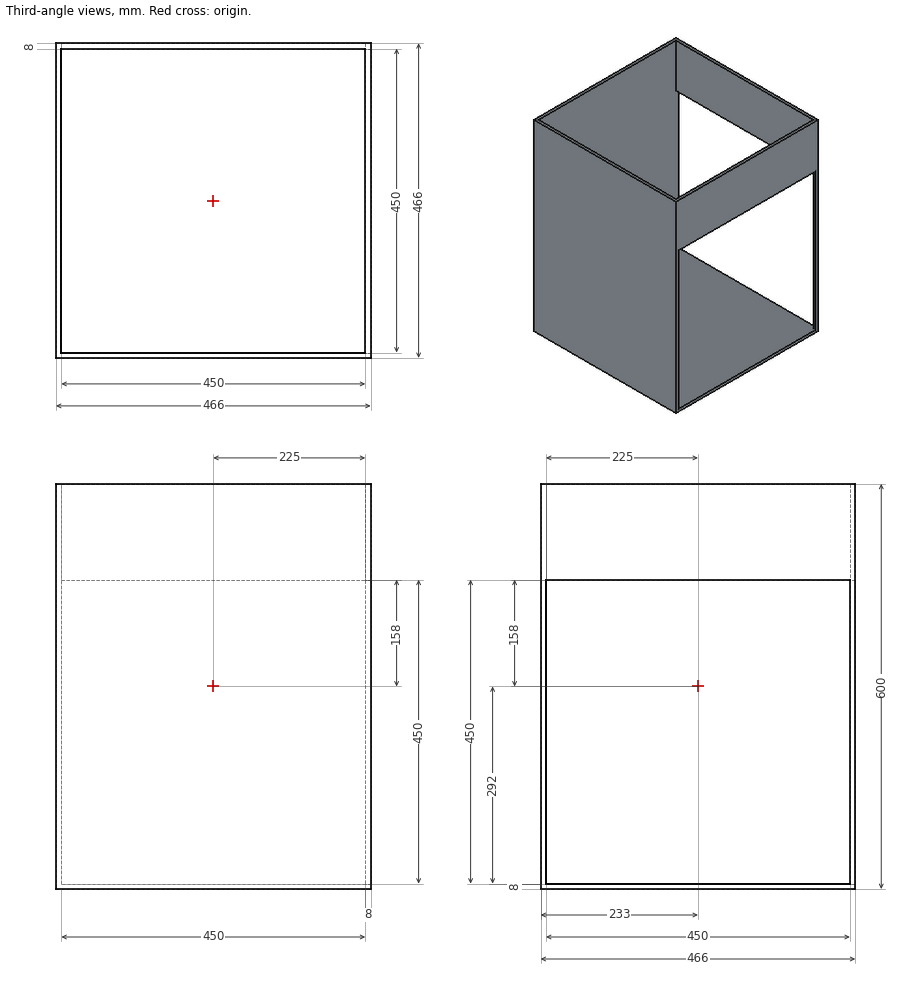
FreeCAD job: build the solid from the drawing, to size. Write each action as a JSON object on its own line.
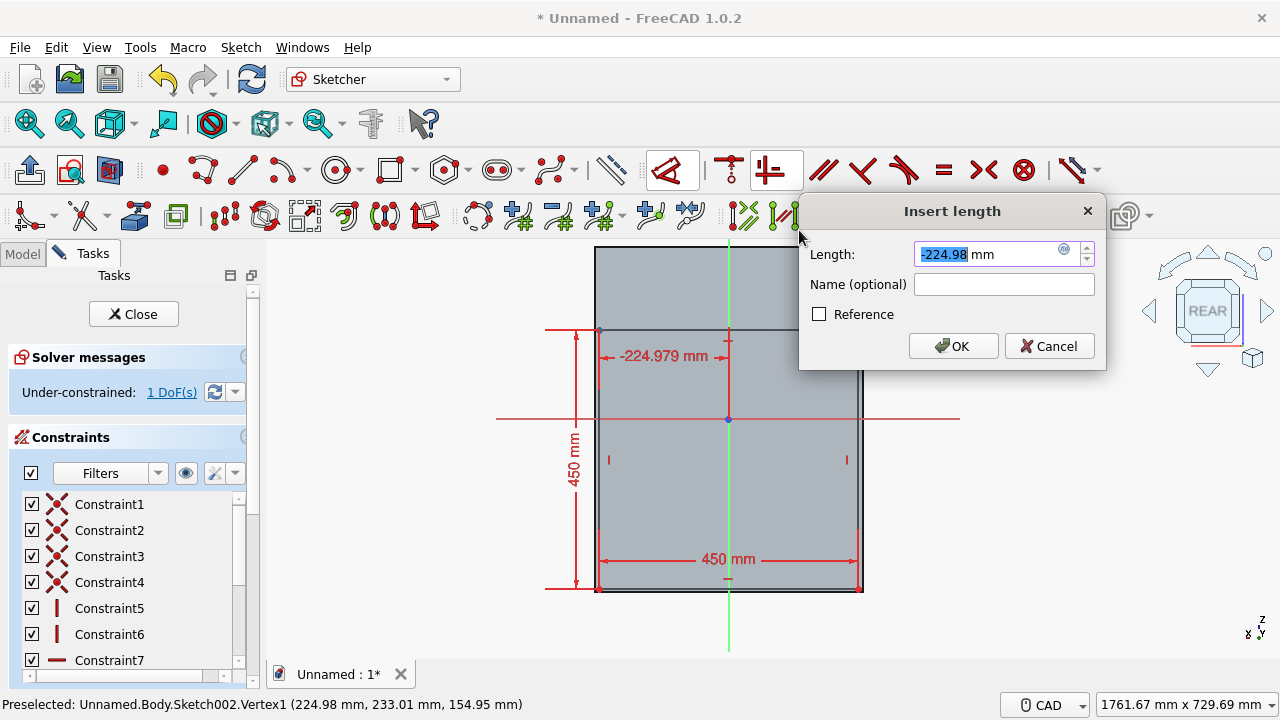
{"action": "type", "text": "-225"}
{"action": "key", "text": "Return"}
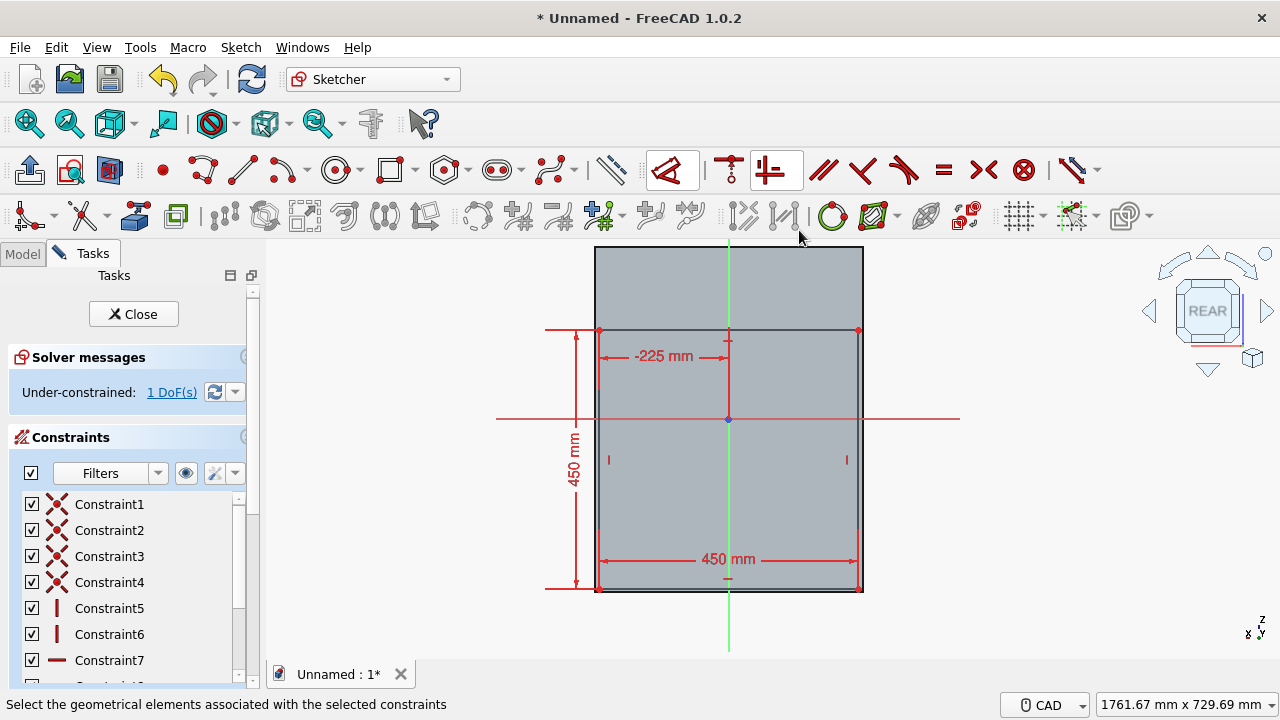
{"action": "left_click", "coordinate": [599, 330]}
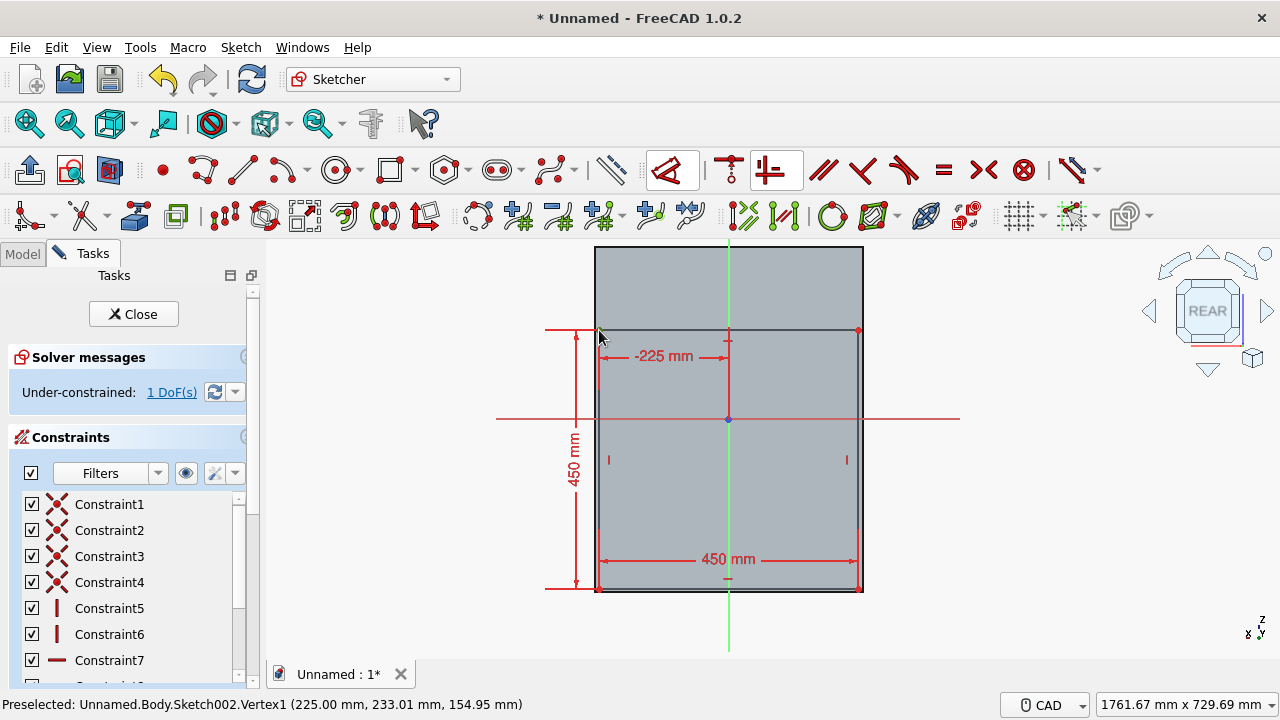
{"action": "key", "text": "i"}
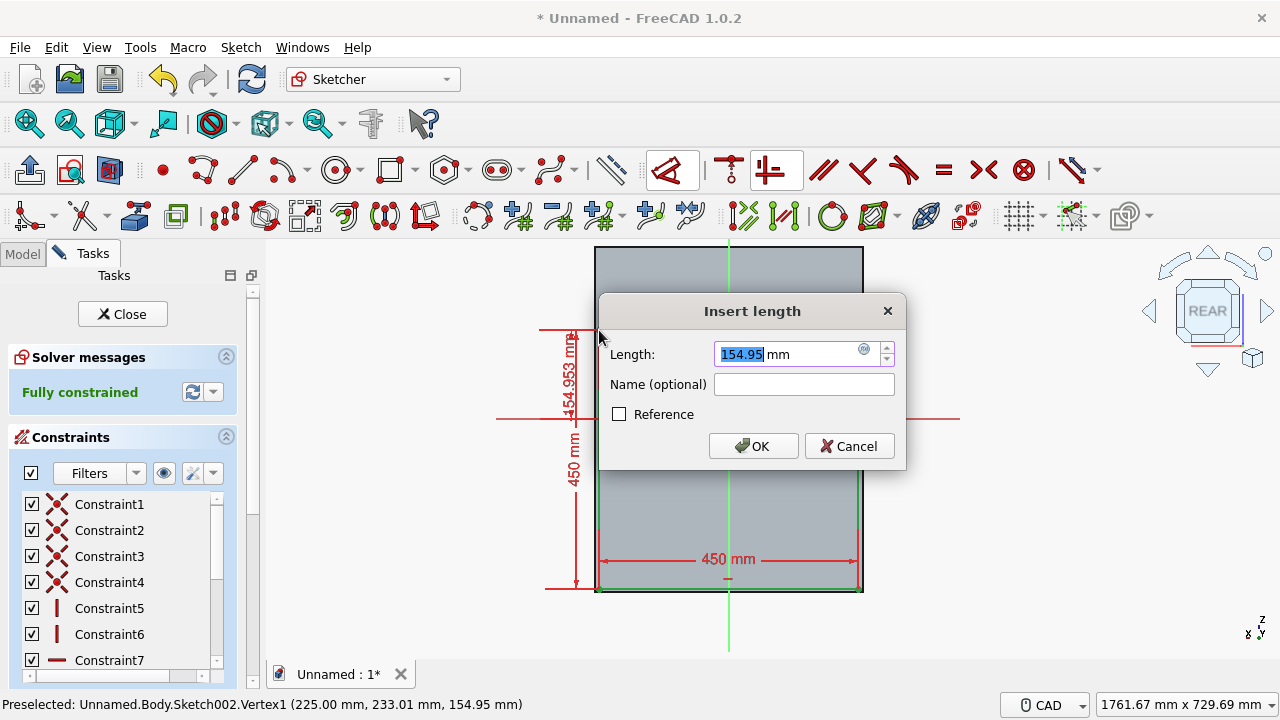
{"action": "type", "text": "158"}
{"action": "key", "text": "Return"}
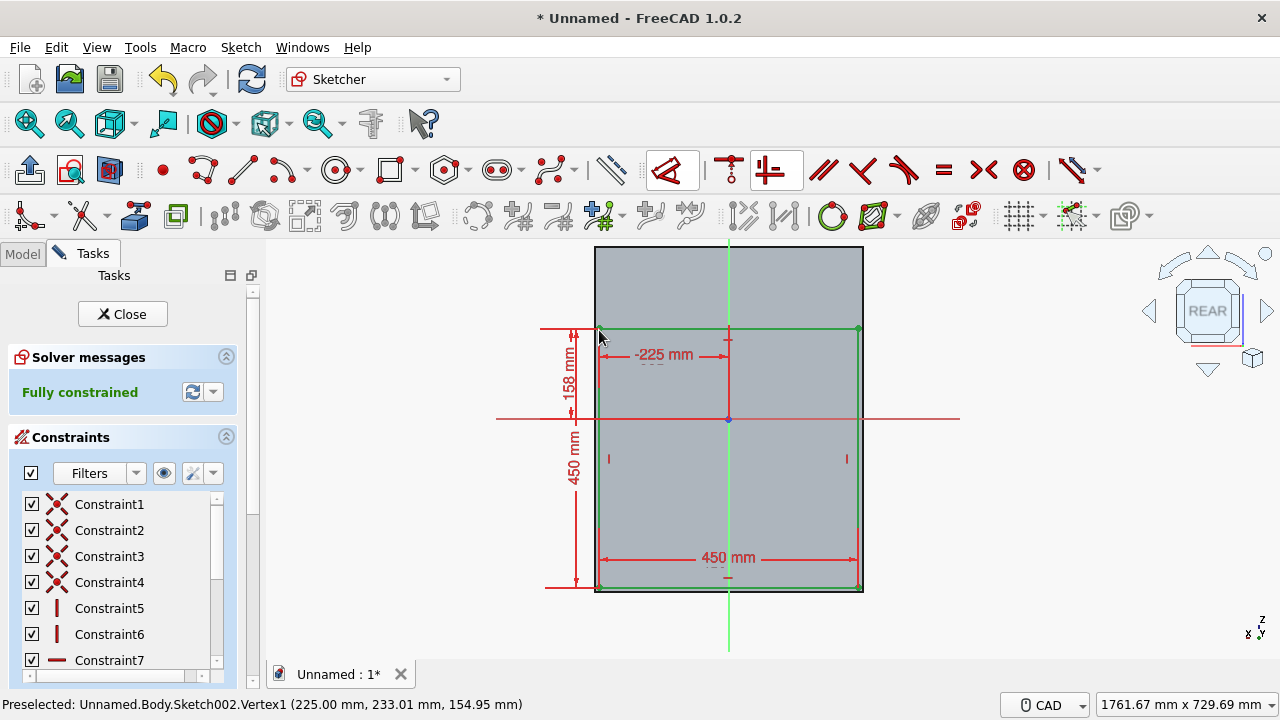
{"action": "left_click", "coordinate": [123, 314]}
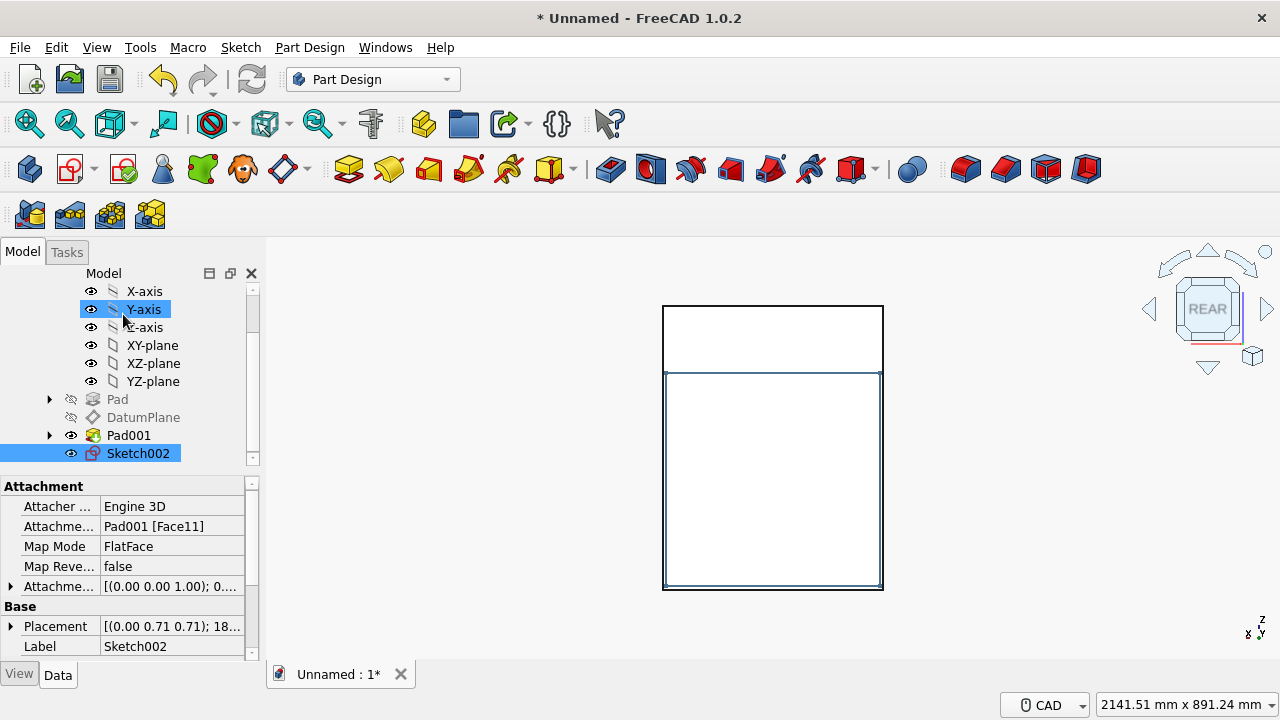
{"action": "left_click", "coordinate": [612, 170]}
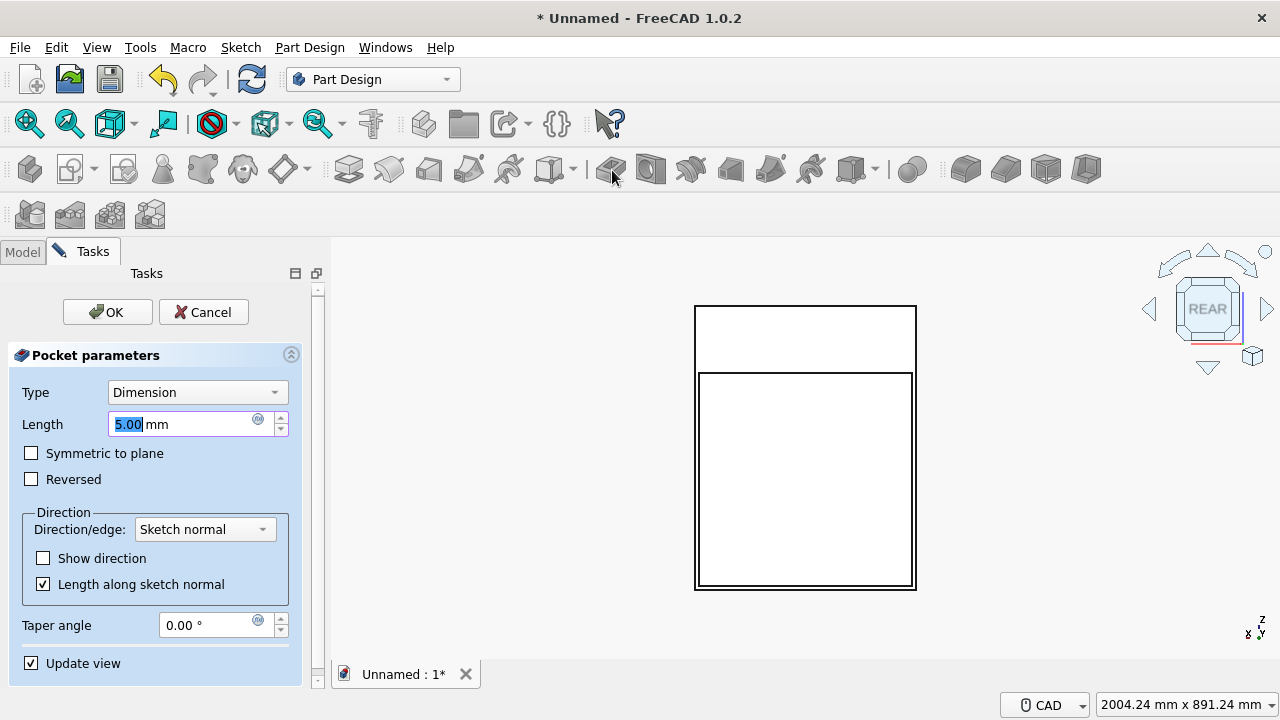
{"action": "type", "text": "8"}
{"action": "key", "text": "Tab"}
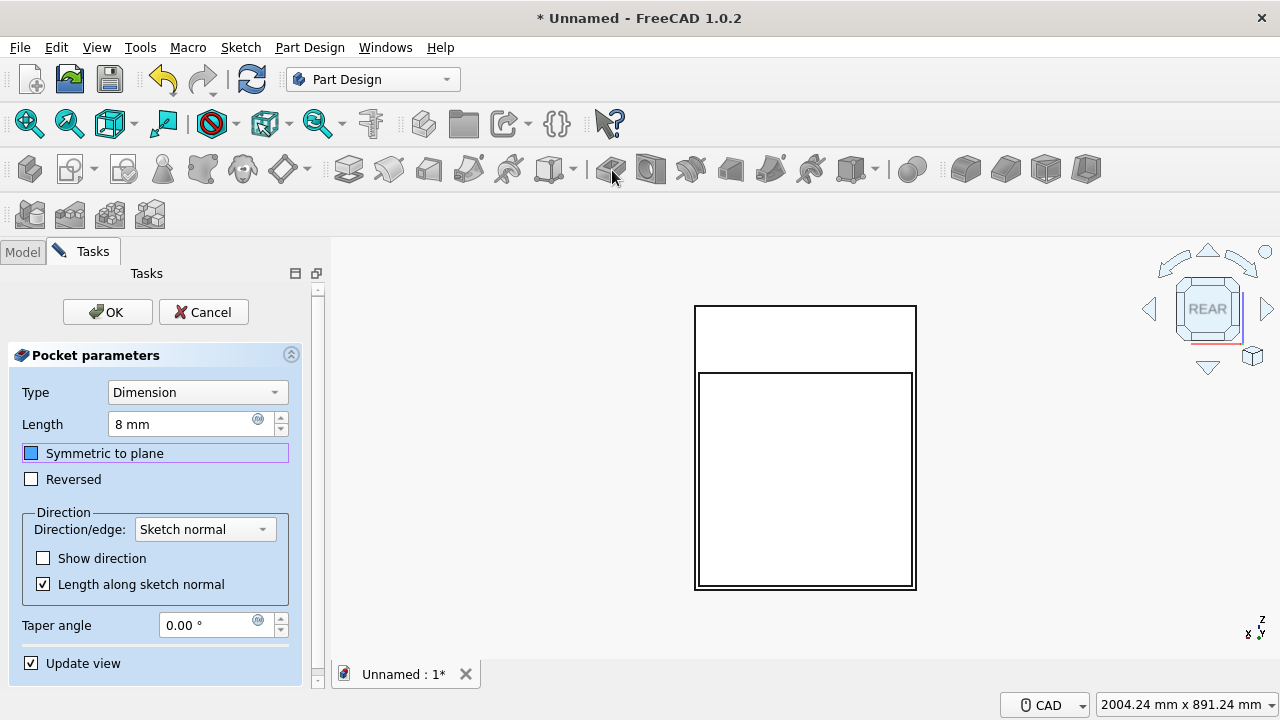
{"action": "left_click", "coordinate": [108, 312]}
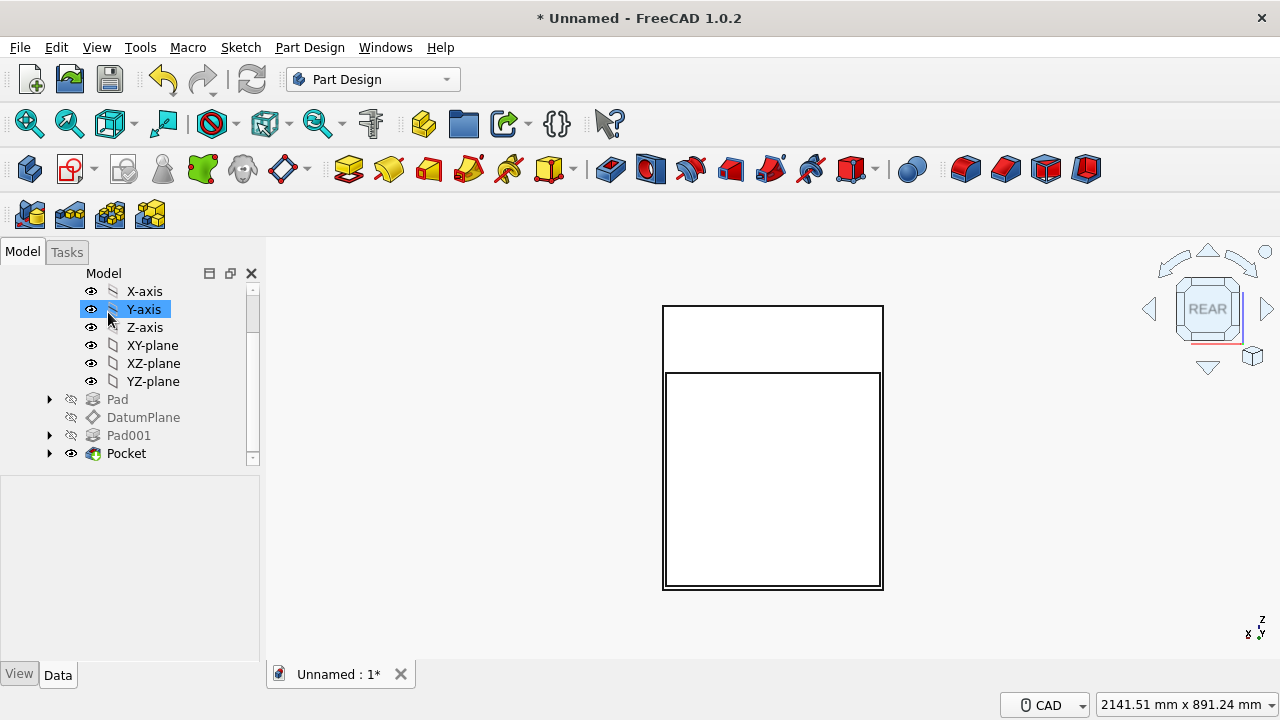
{"action": "key", "text": "0"}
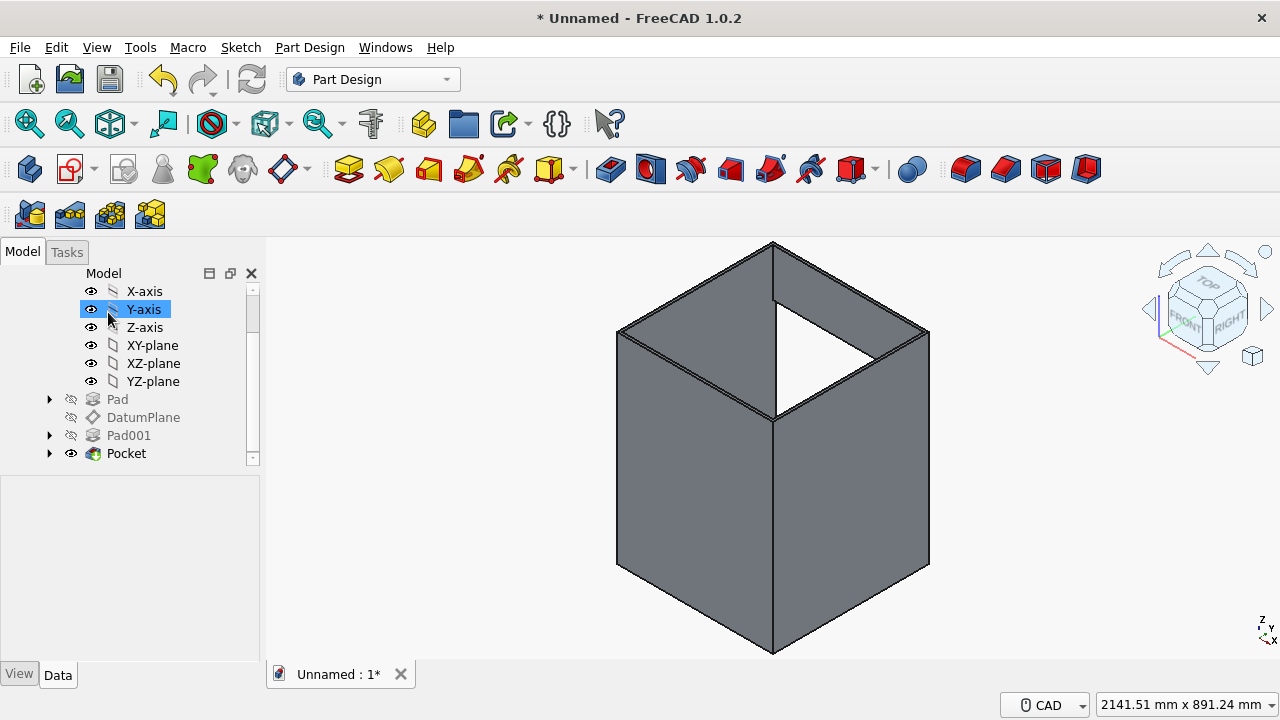
{"action": "left_click", "coordinate": [851, 492]}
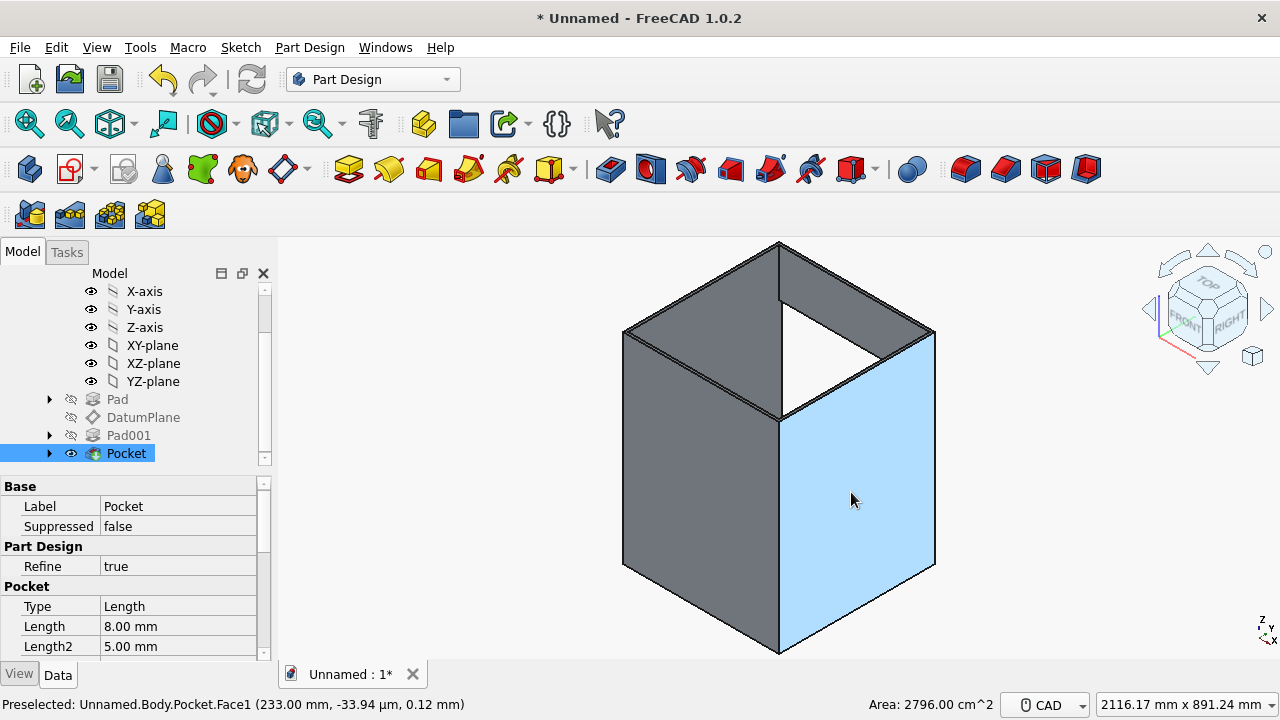
{"action": "left_click", "coordinate": [70, 170]}